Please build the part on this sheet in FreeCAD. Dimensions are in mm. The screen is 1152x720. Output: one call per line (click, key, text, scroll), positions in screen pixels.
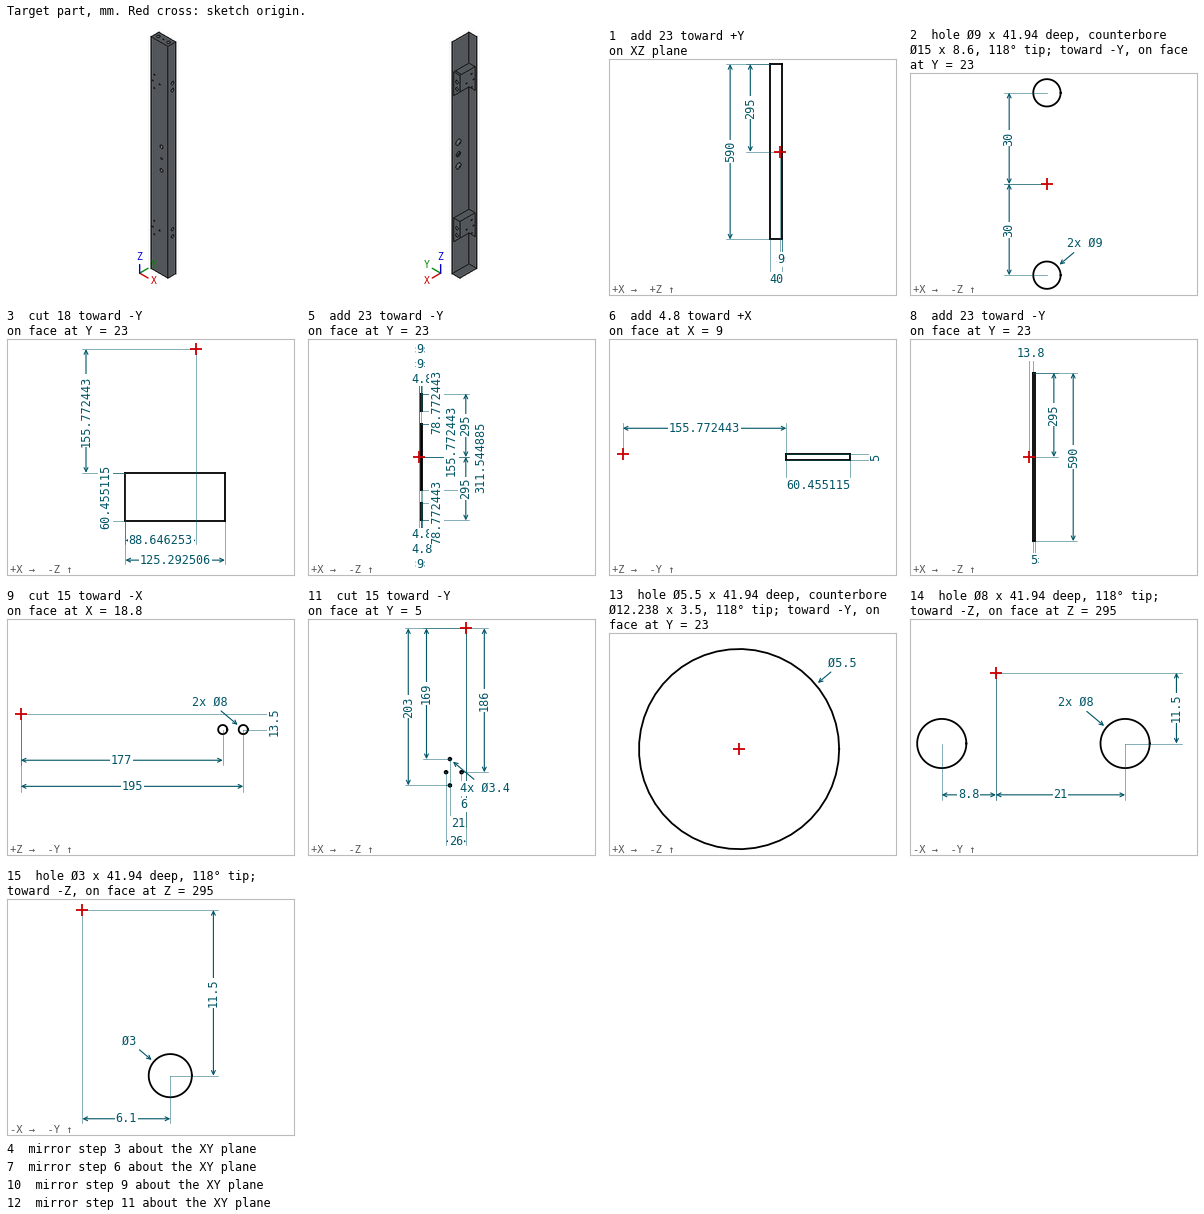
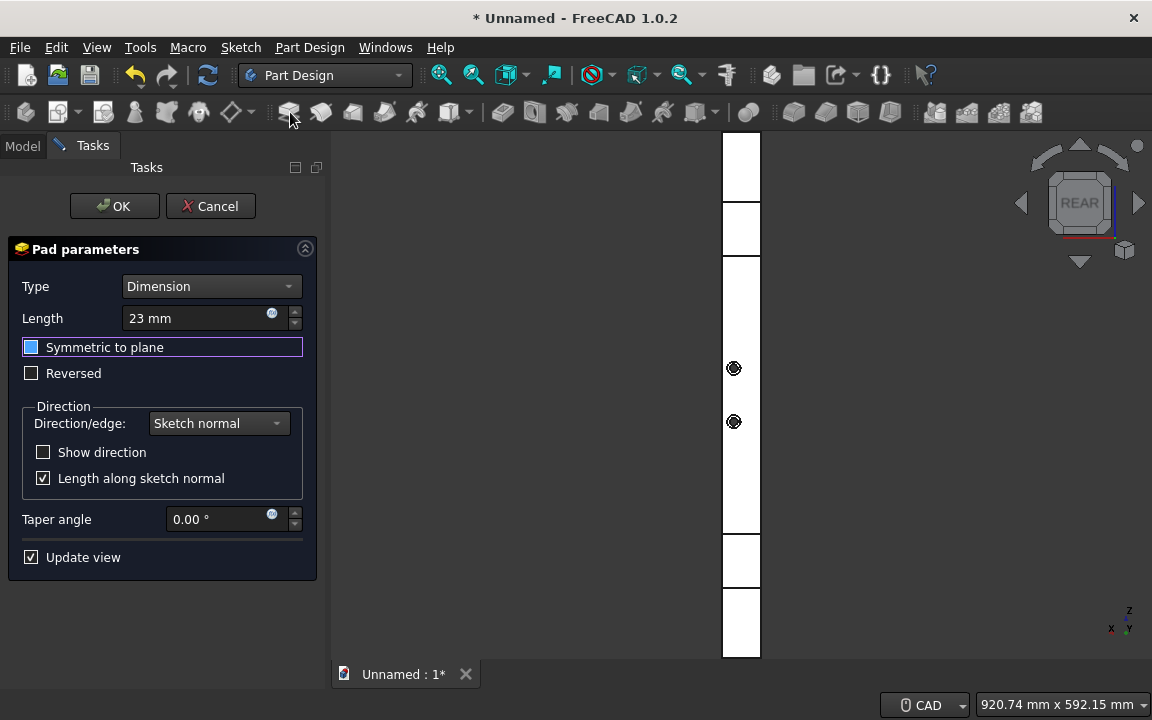
click(30, 373)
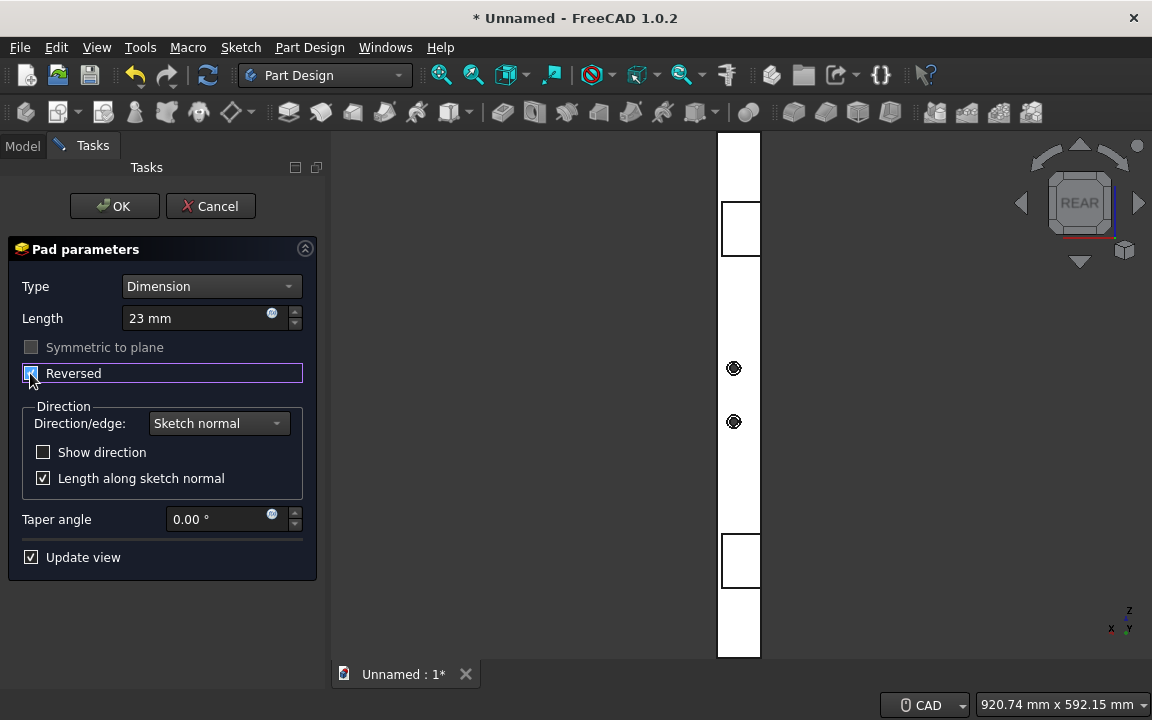
click(115, 206)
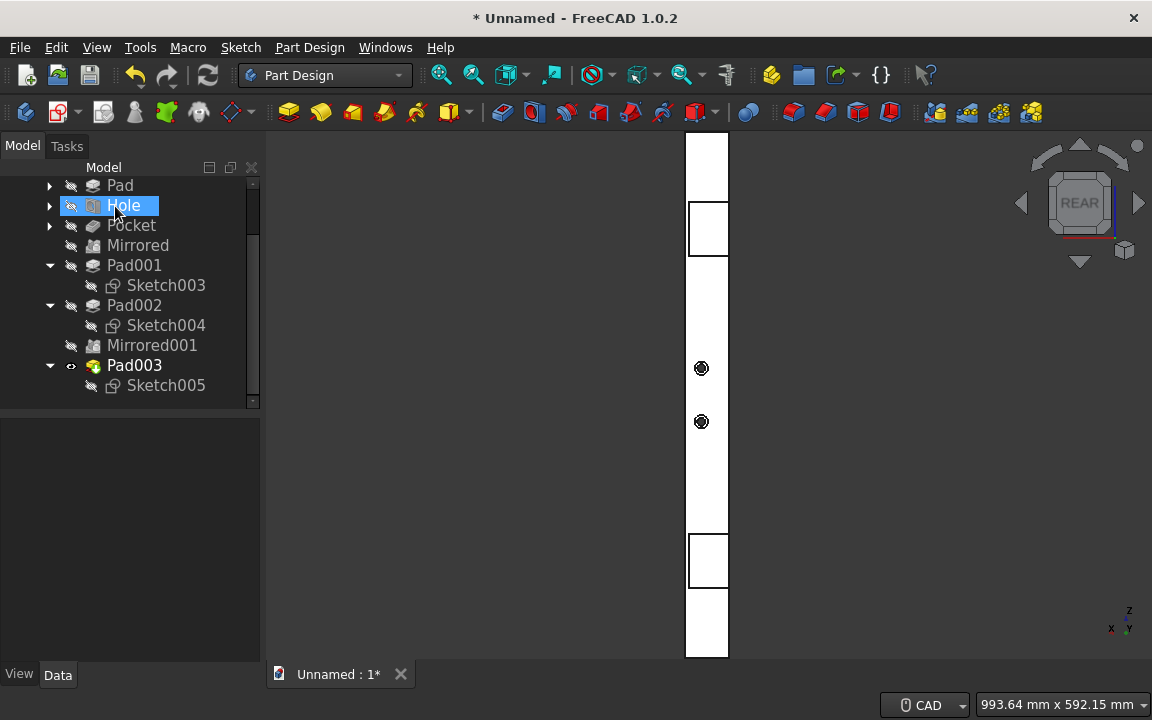
key(0)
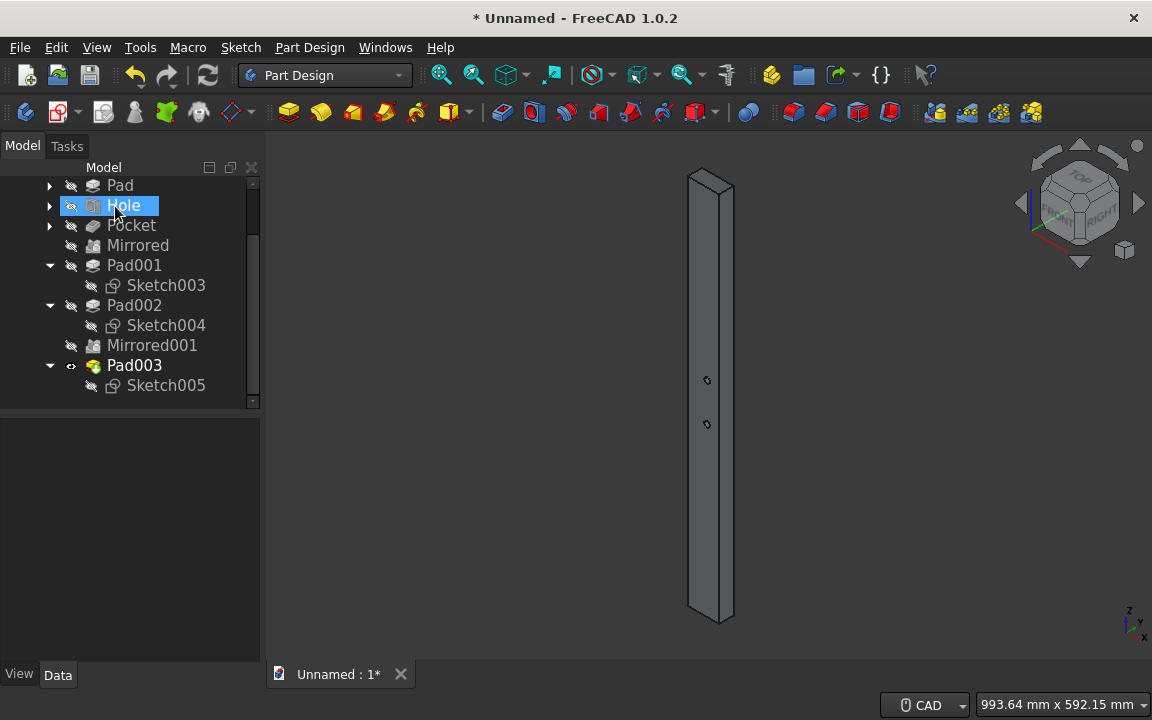
click(728, 219)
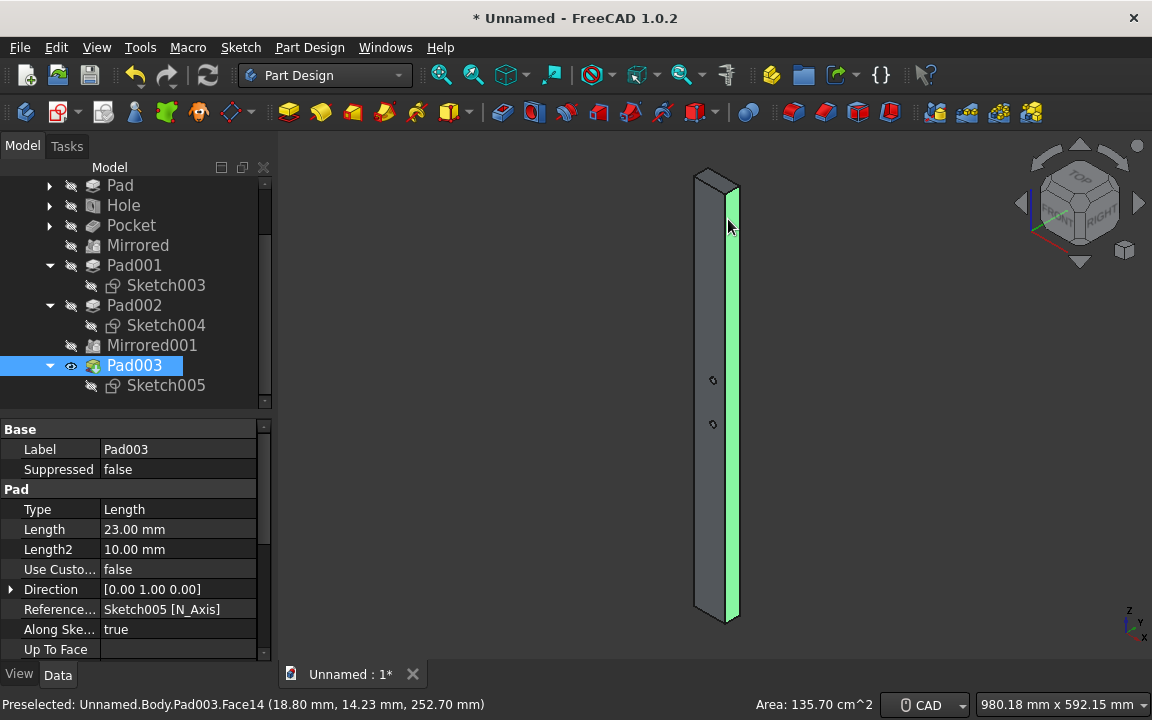
click(58, 112)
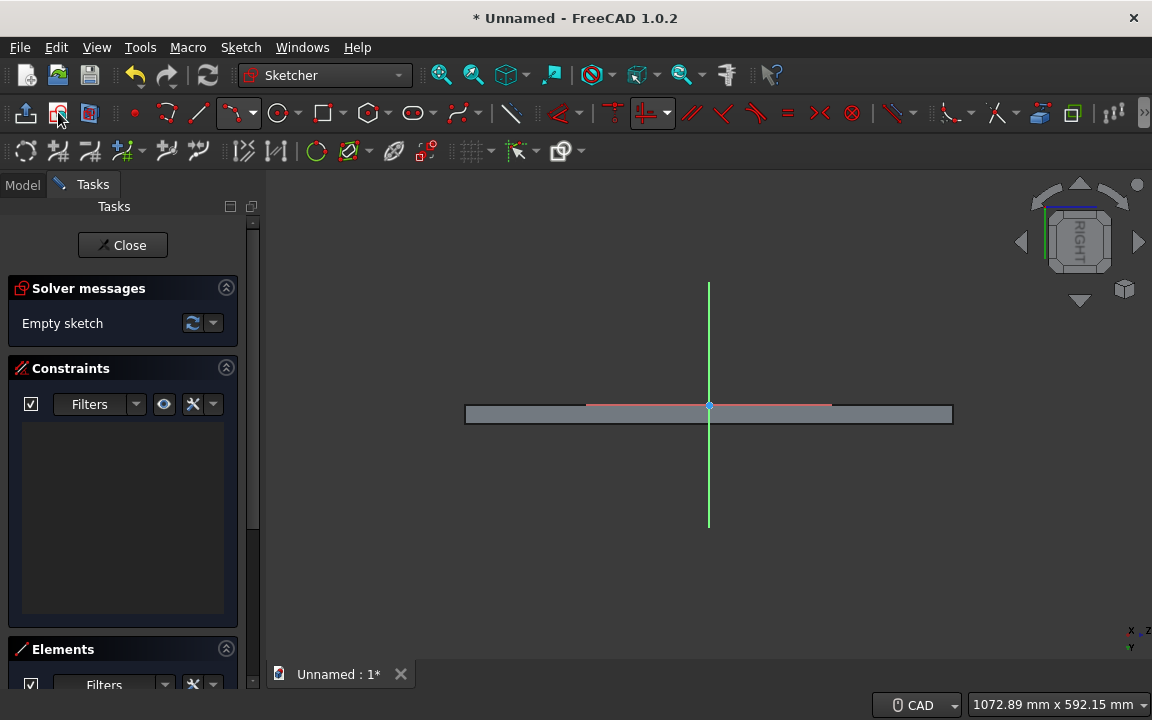
scroll(874, 416, up, 15)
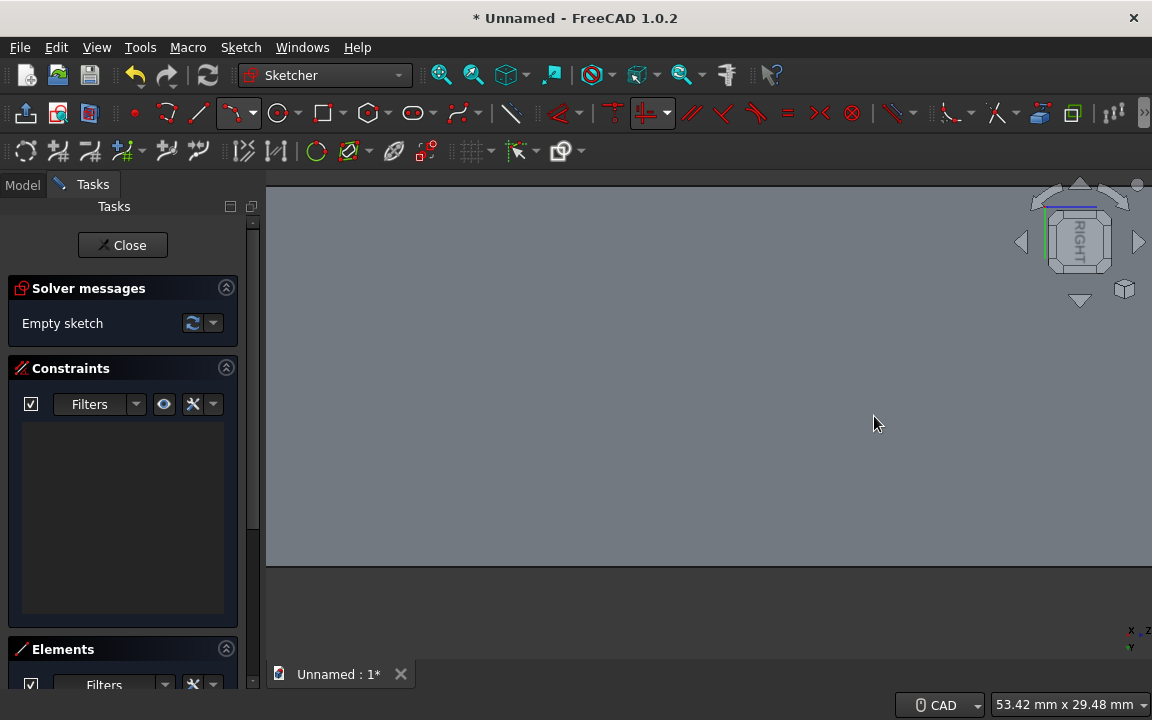
click(278, 114)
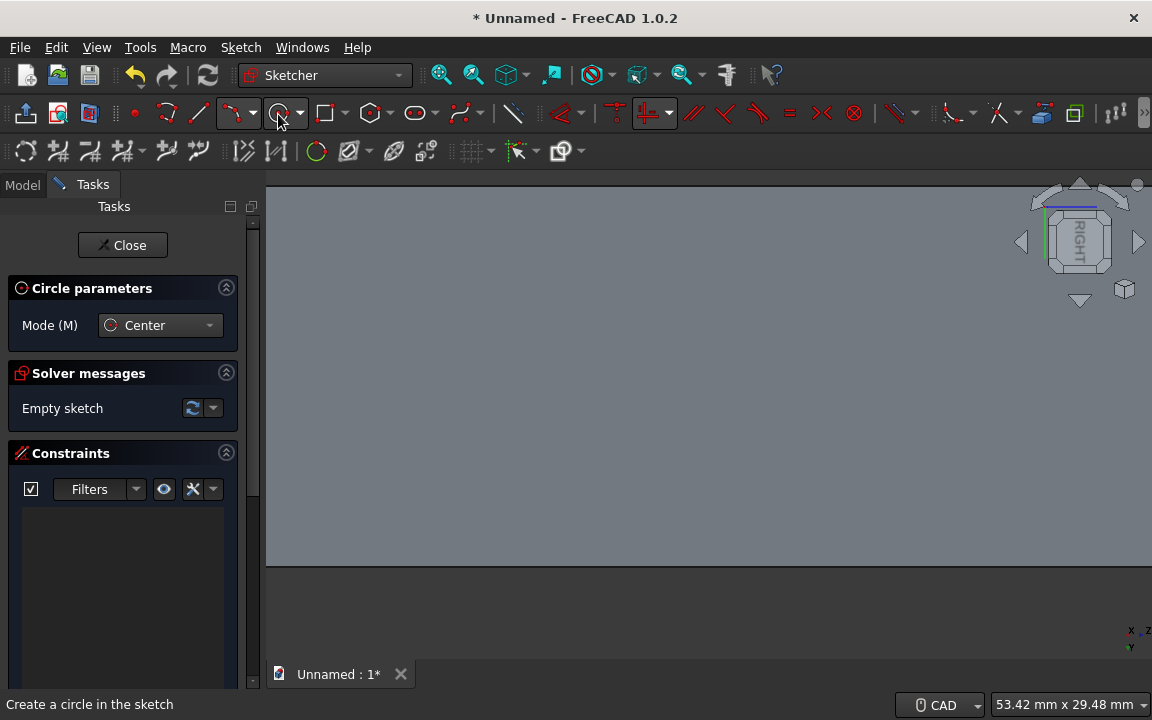
click(781, 409)
click(828, 363)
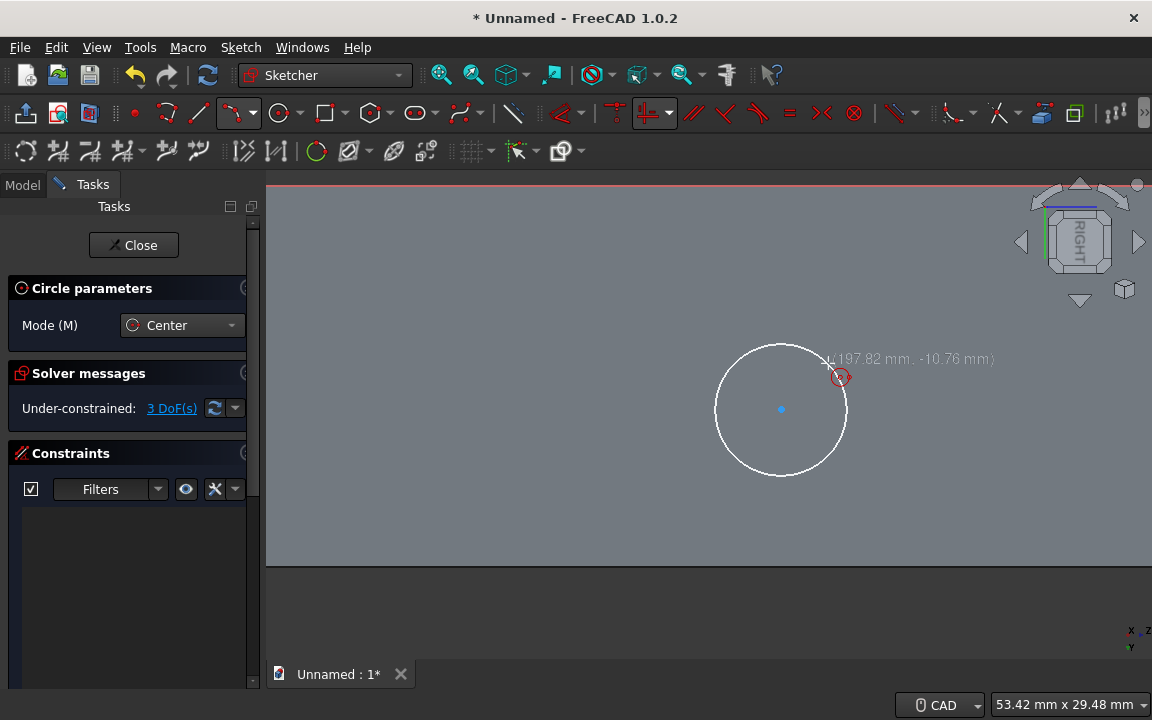
click(483, 409)
click(530, 363)
key(Escape)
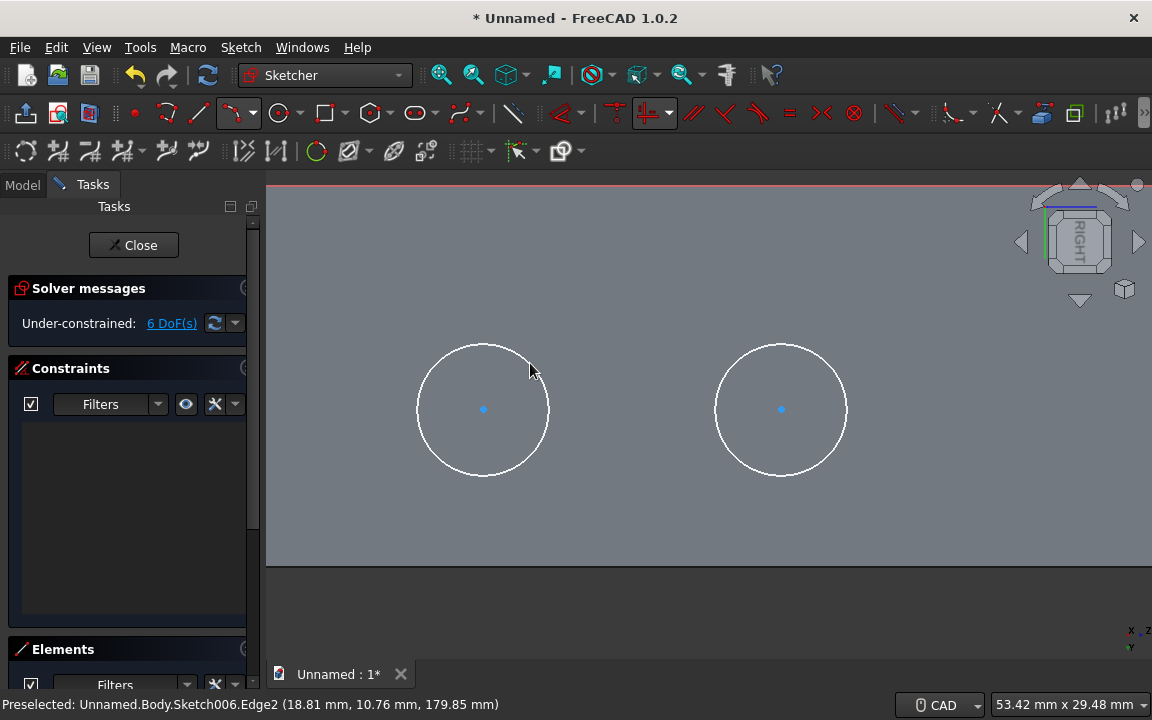
click(827, 363)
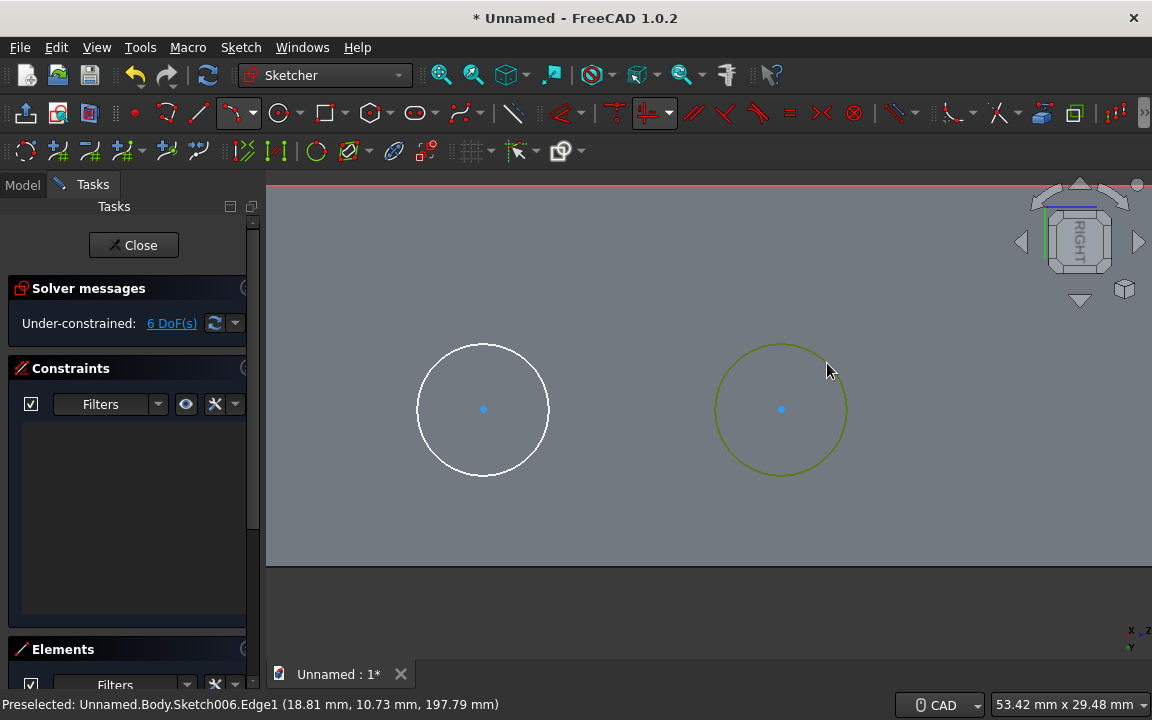
click(529, 363)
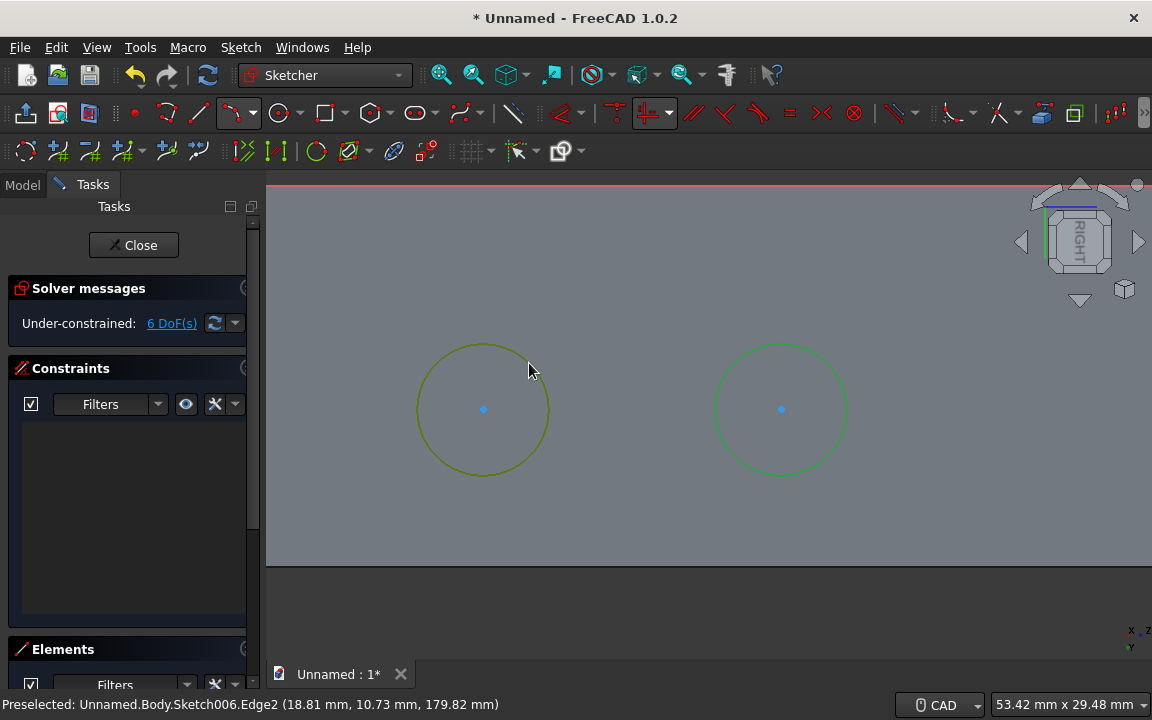
click(790, 114)